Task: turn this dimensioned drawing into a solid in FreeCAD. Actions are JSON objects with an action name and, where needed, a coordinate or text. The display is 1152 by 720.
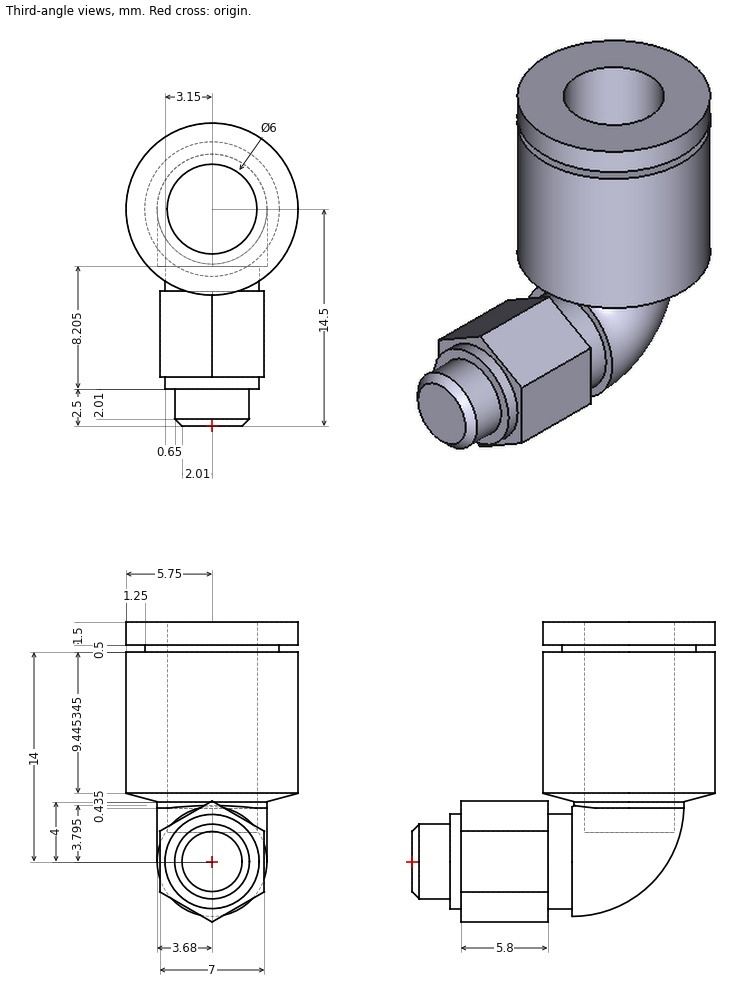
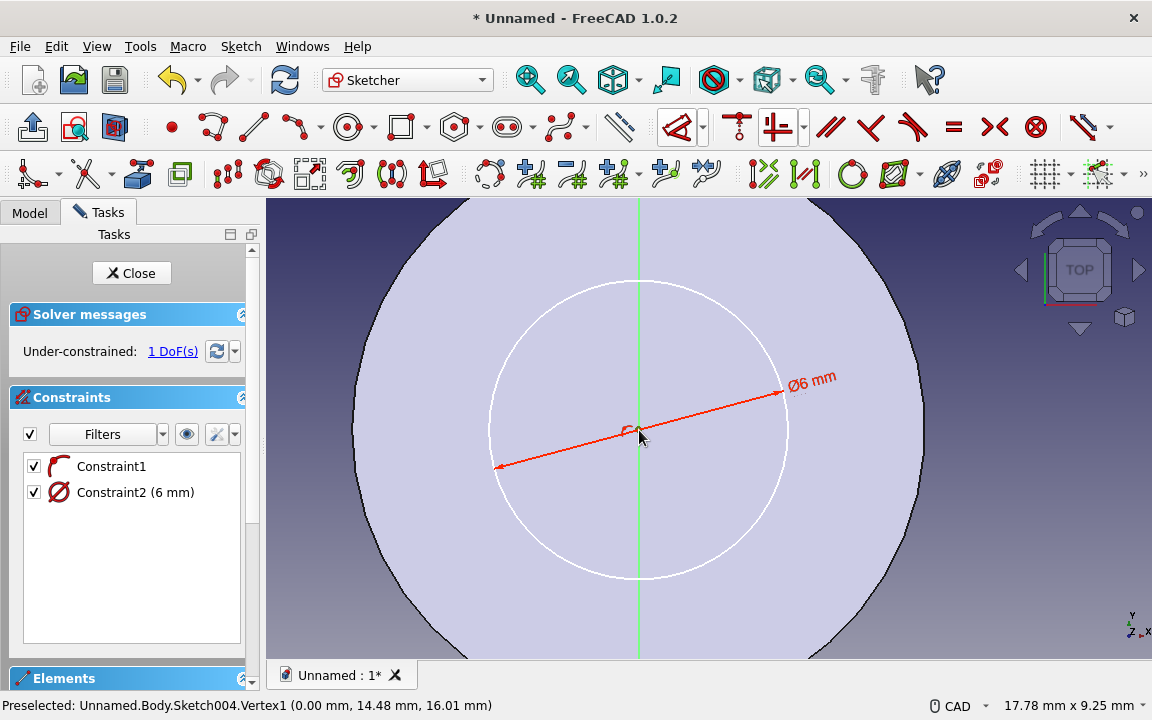
{"action": "key", "text": "i"}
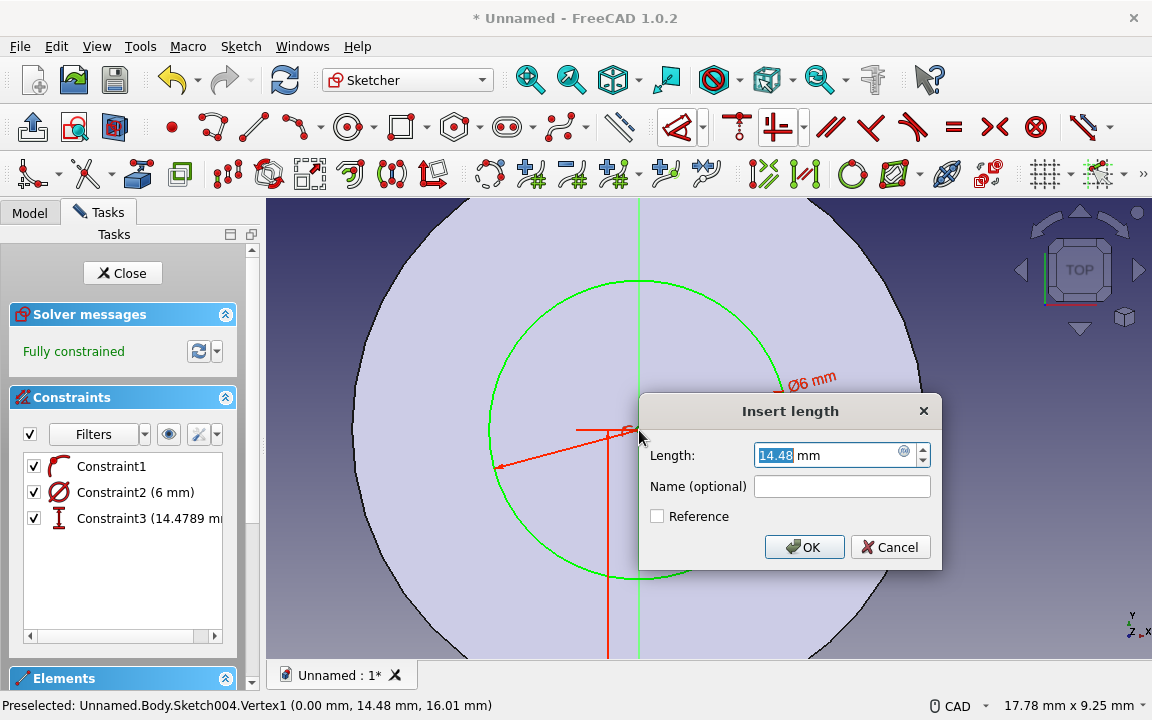
{"action": "type", "text": "14.5"}
{"action": "key", "text": "Return"}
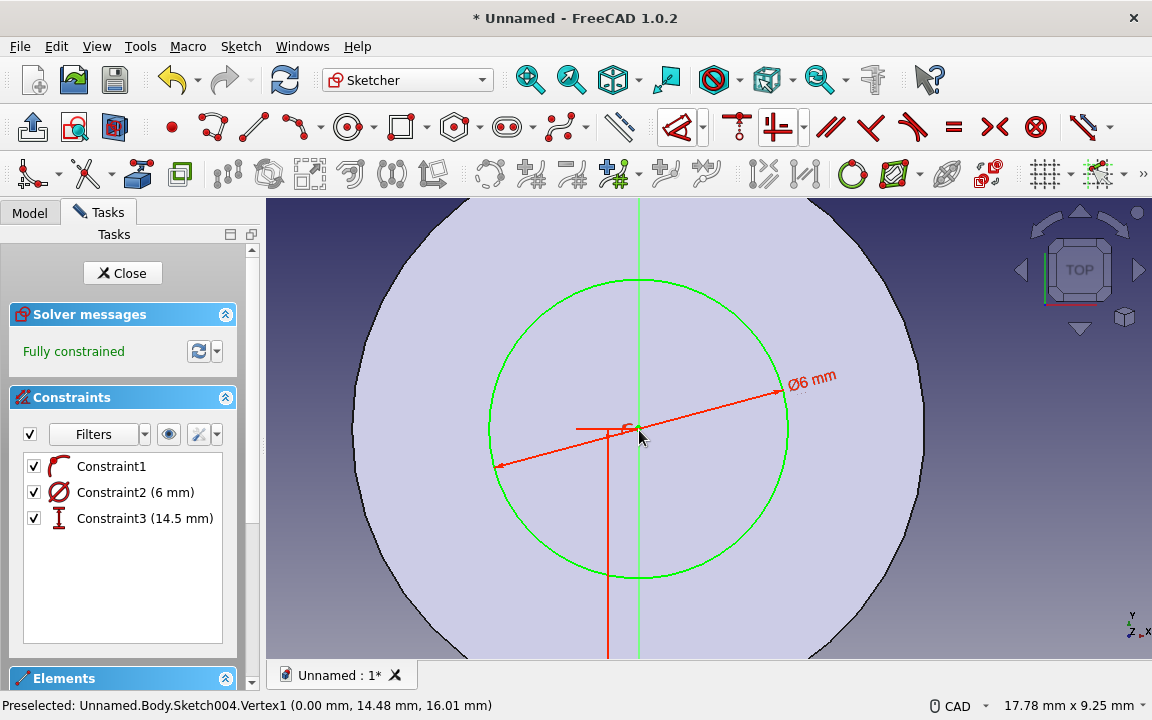
{"action": "left_click", "coordinate": [123, 273]}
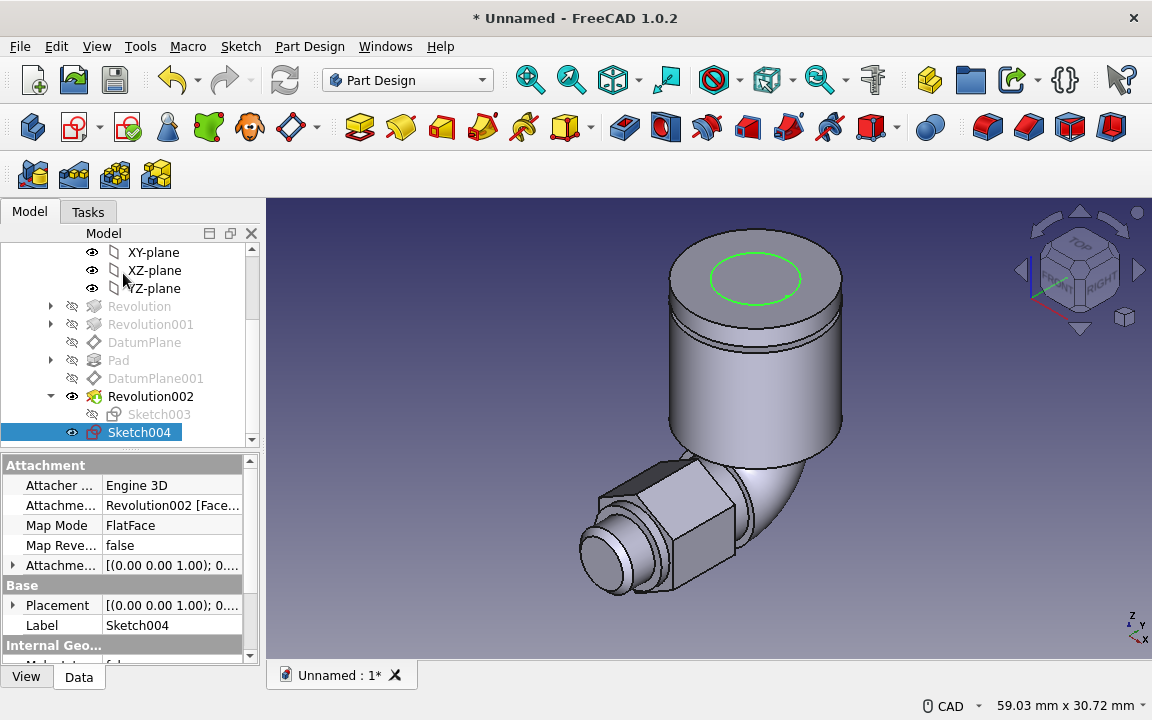
{"action": "left_click", "coordinate": [625, 128]}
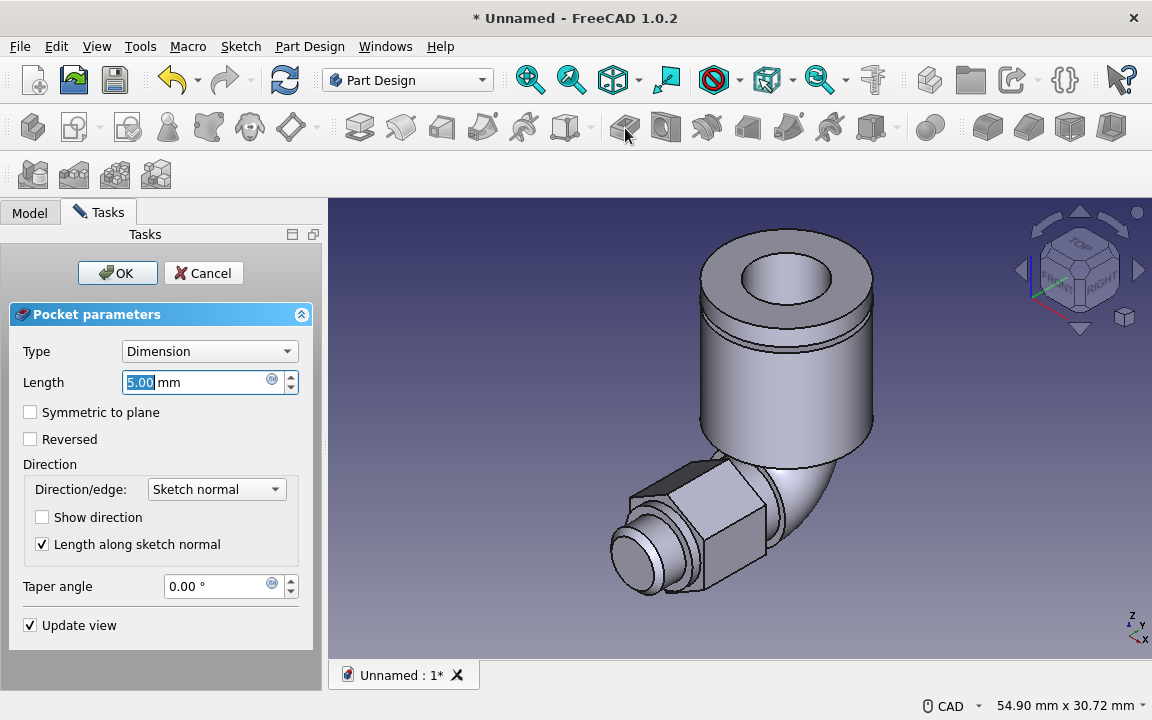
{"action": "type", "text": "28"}
{"action": "key", "text": "Tab"}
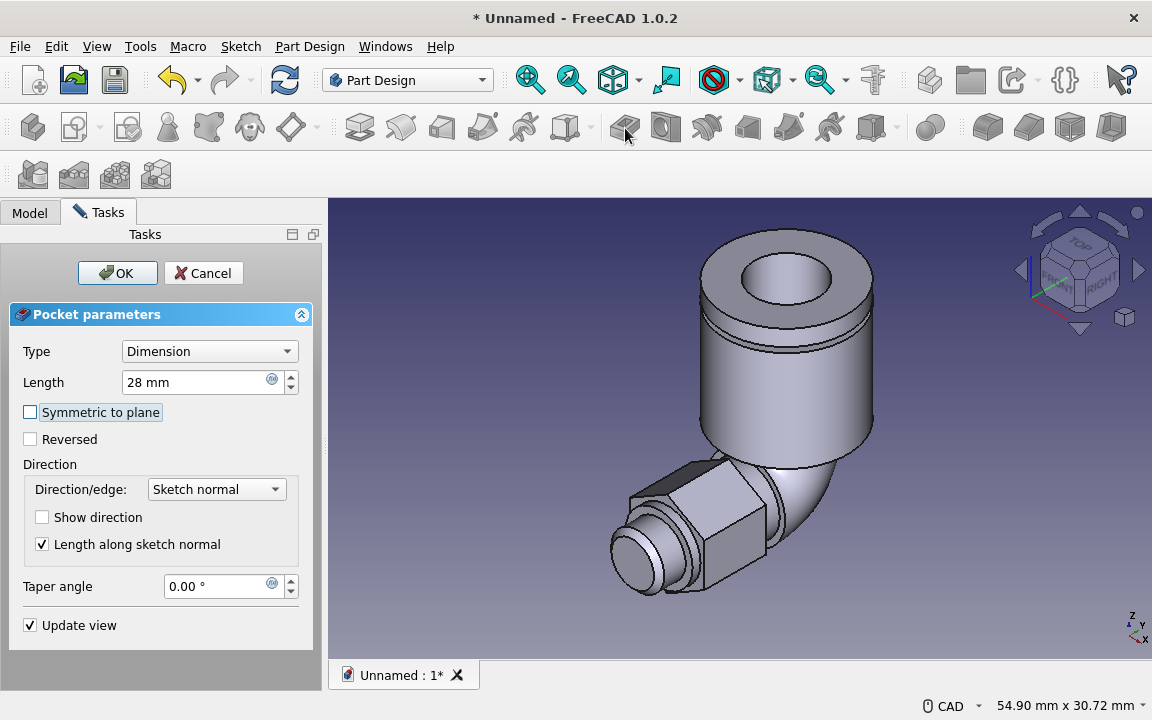
{"action": "left_click", "coordinate": [31, 412]}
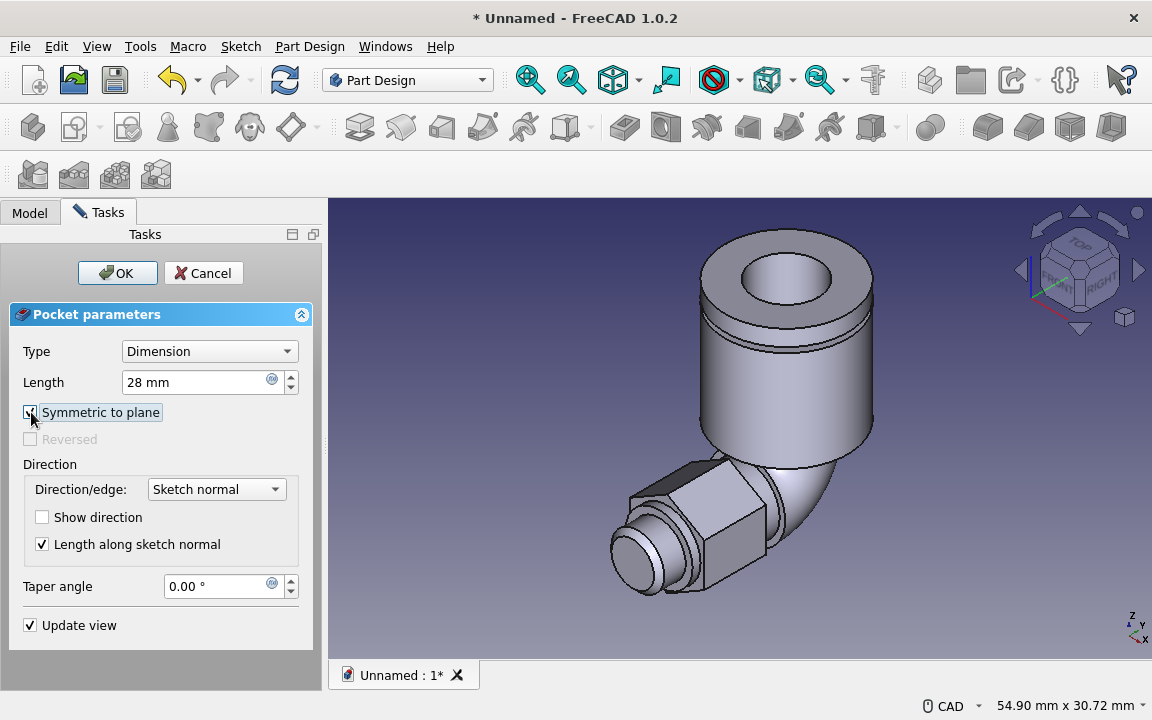
{"action": "left_click", "coordinate": [118, 273]}